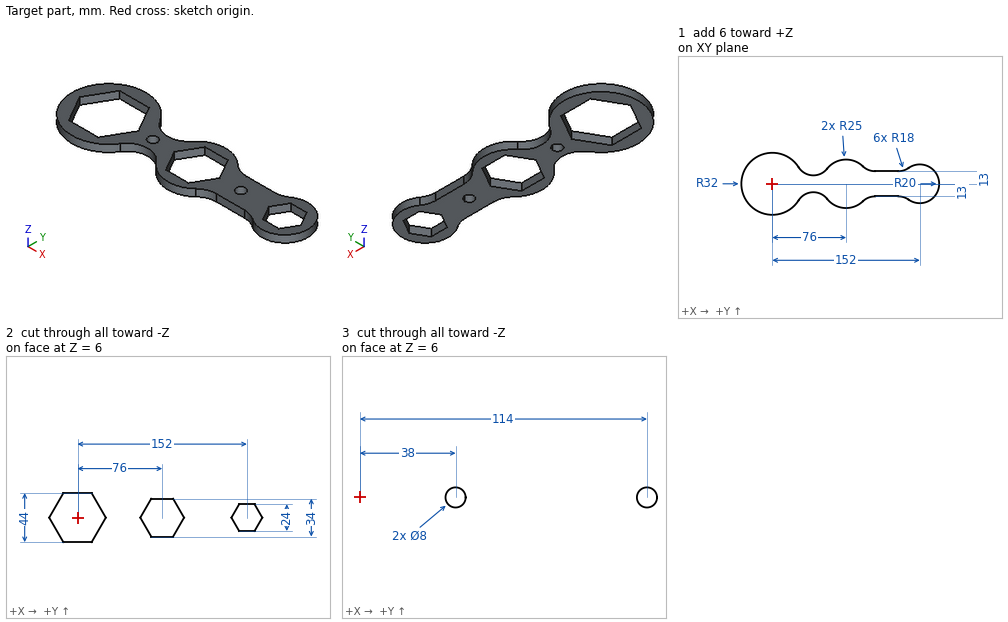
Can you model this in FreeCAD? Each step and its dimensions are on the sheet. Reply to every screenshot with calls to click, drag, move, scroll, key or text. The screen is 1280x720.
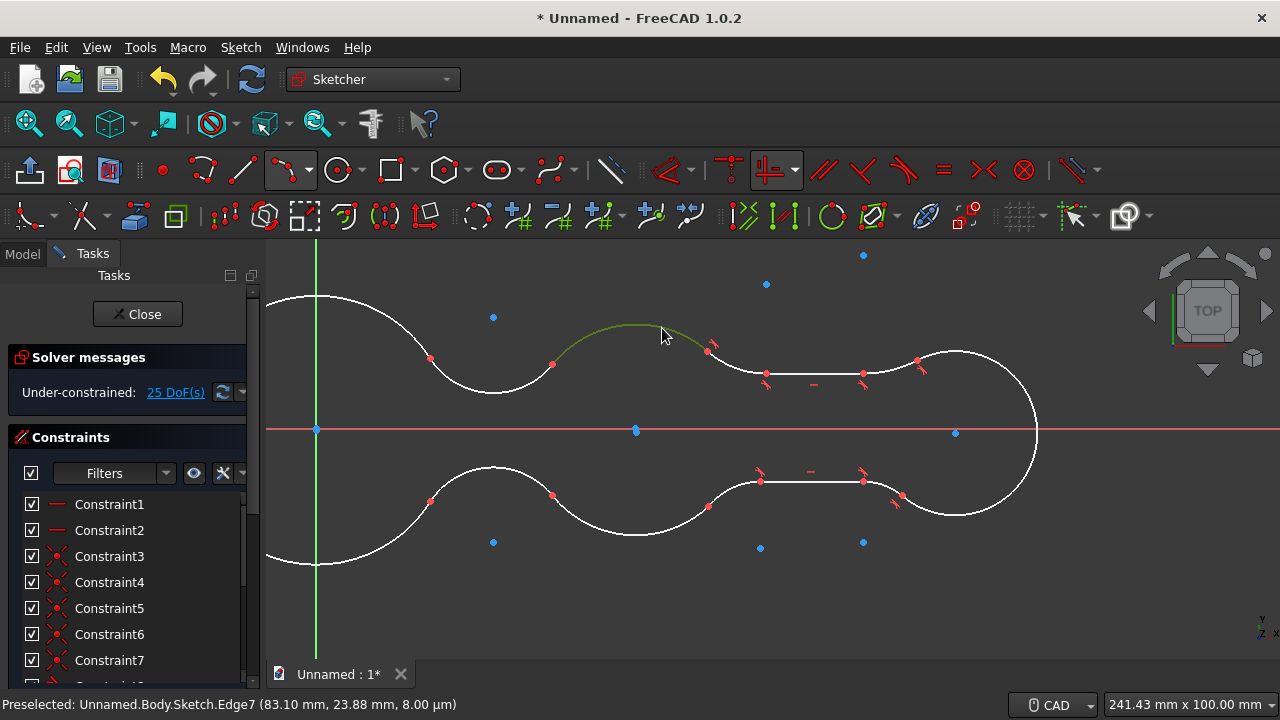
click(462, 386)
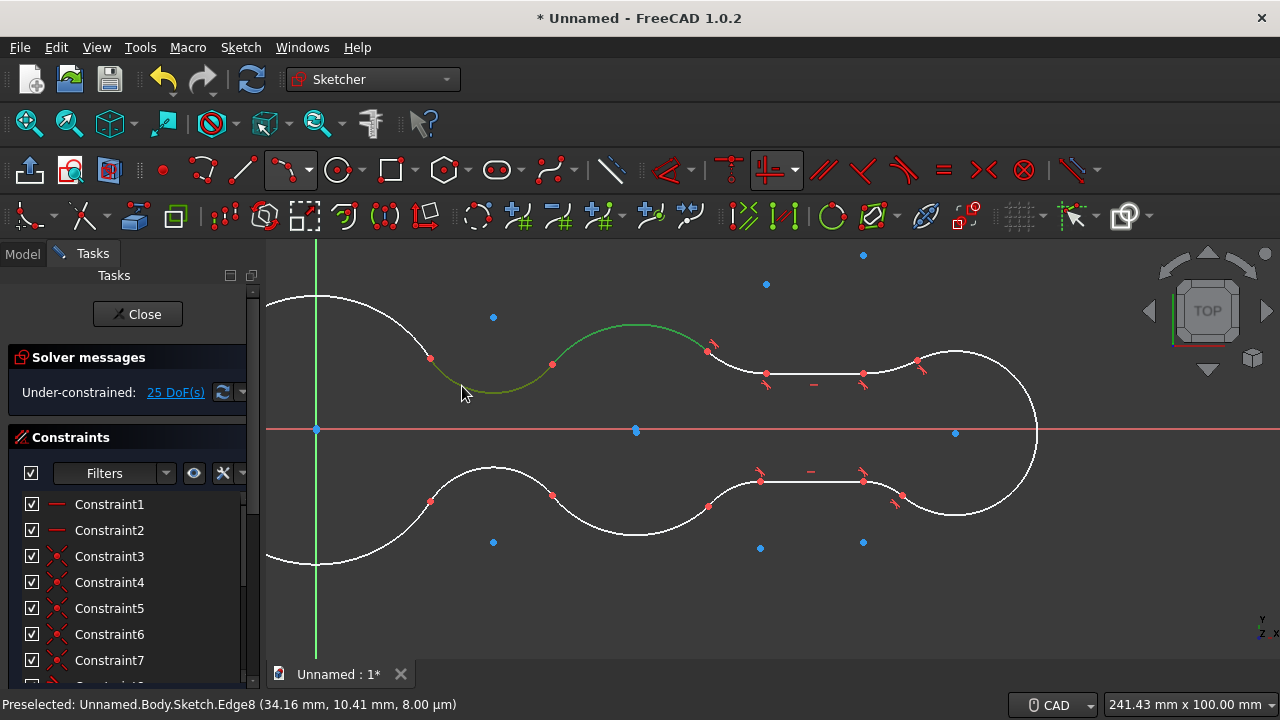
click(904, 170)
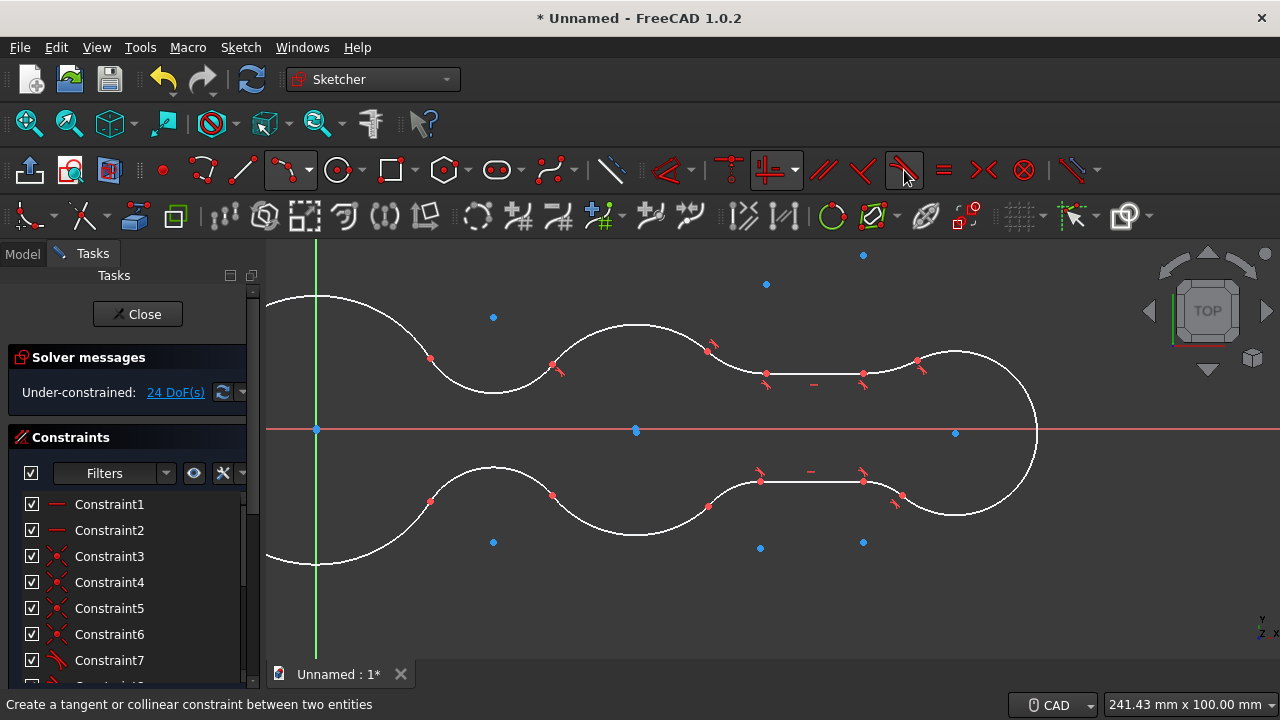
click(462, 386)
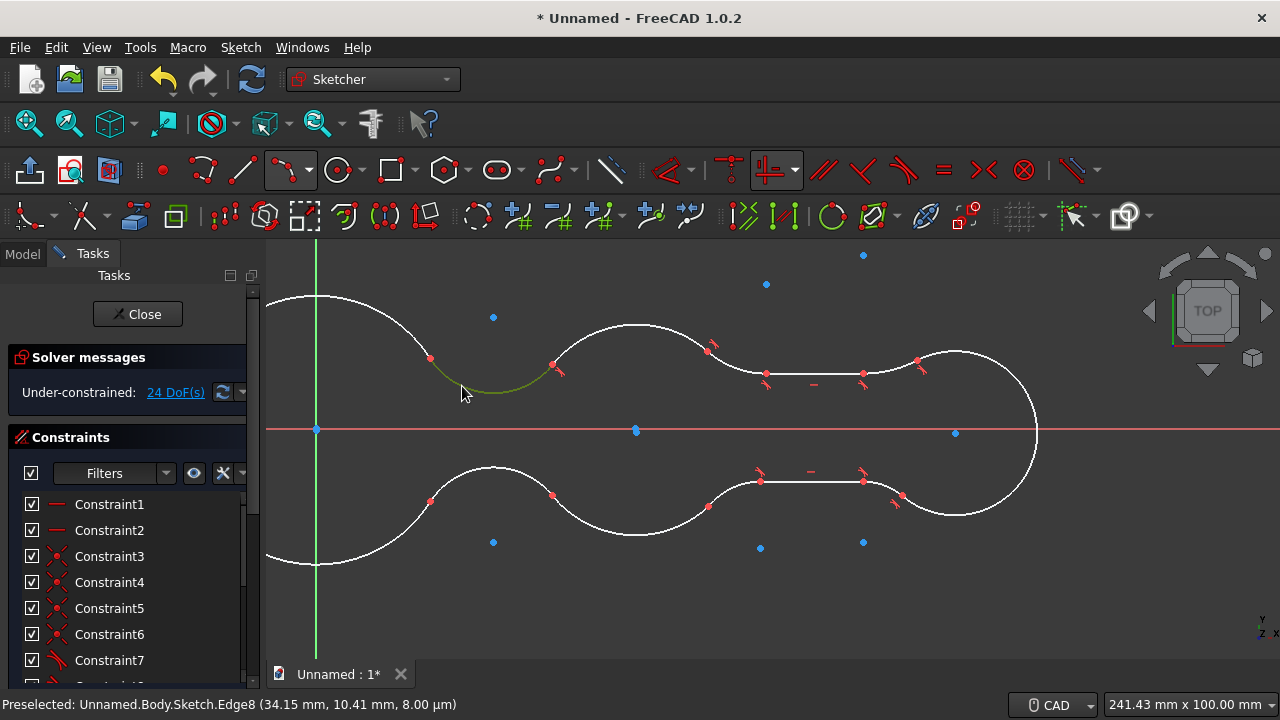
click(313, 296)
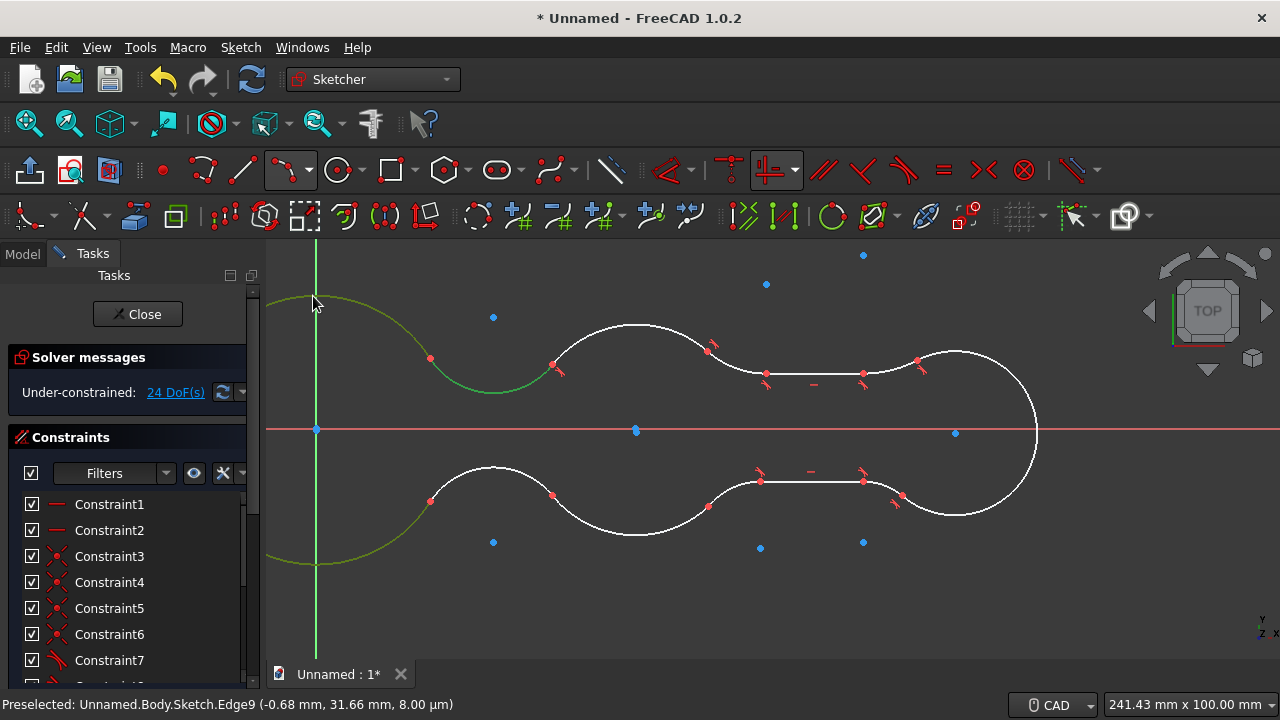
click(904, 170)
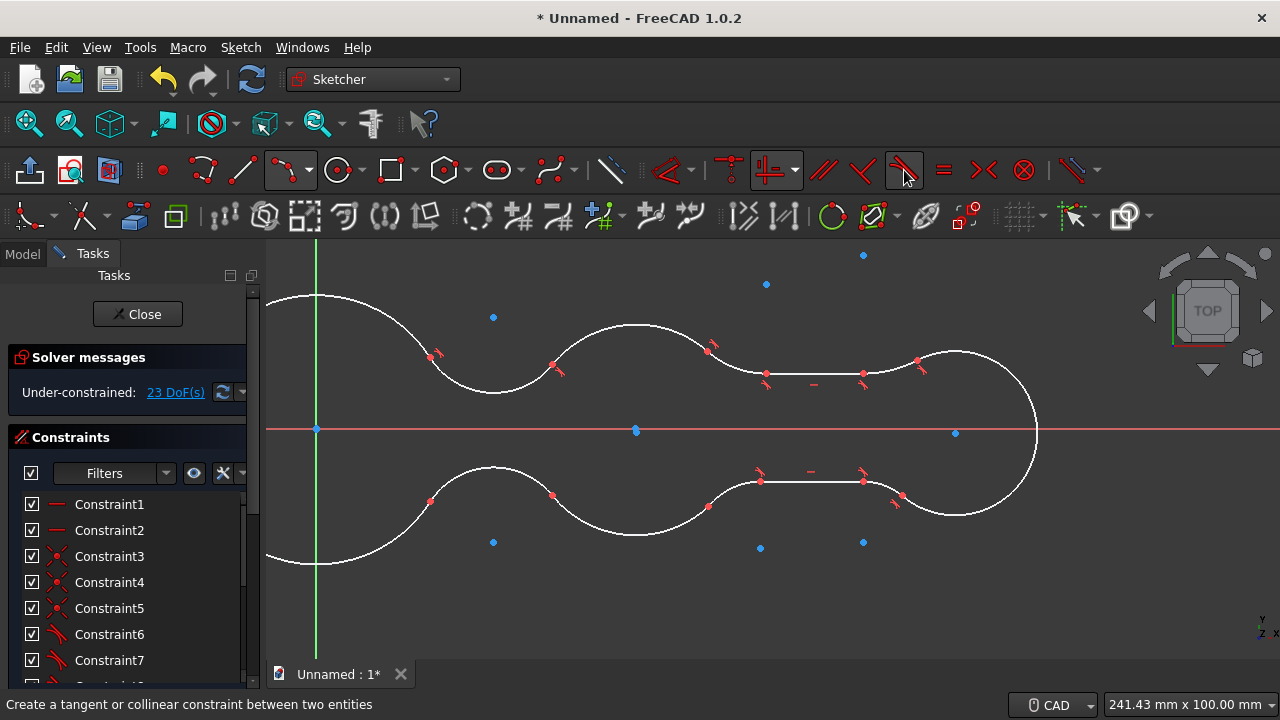
click(313, 295)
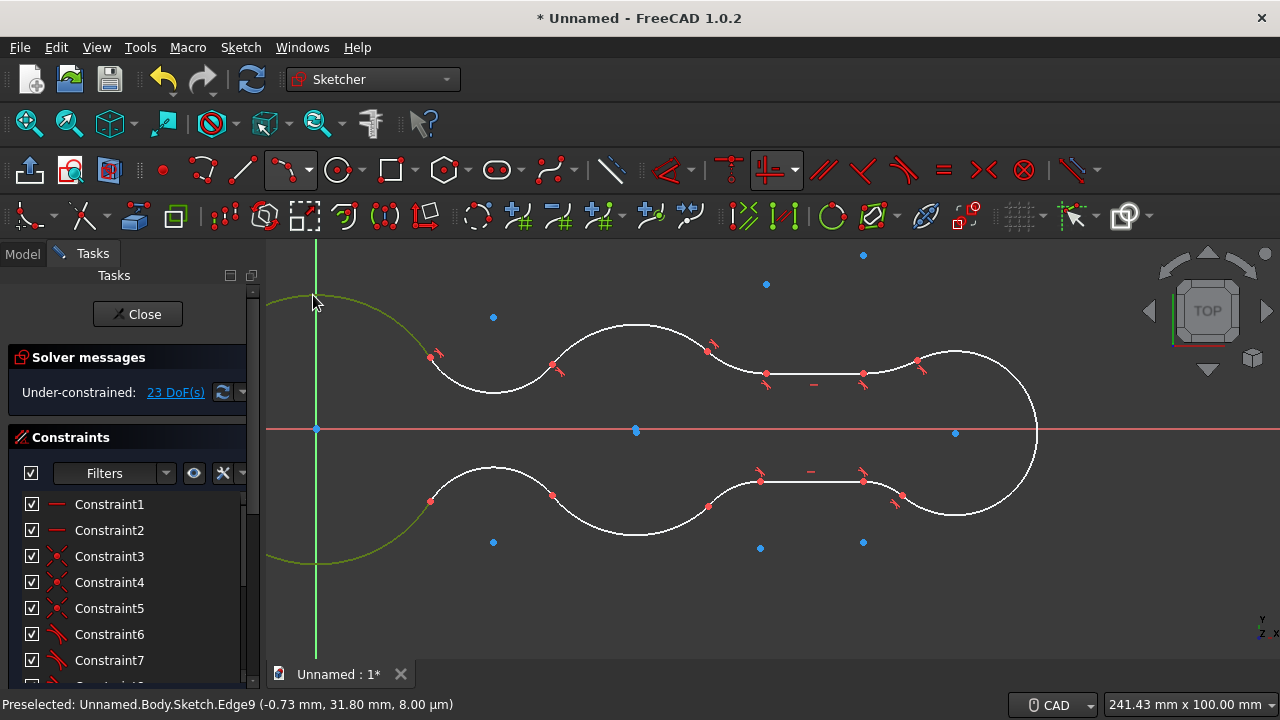
click(518, 472)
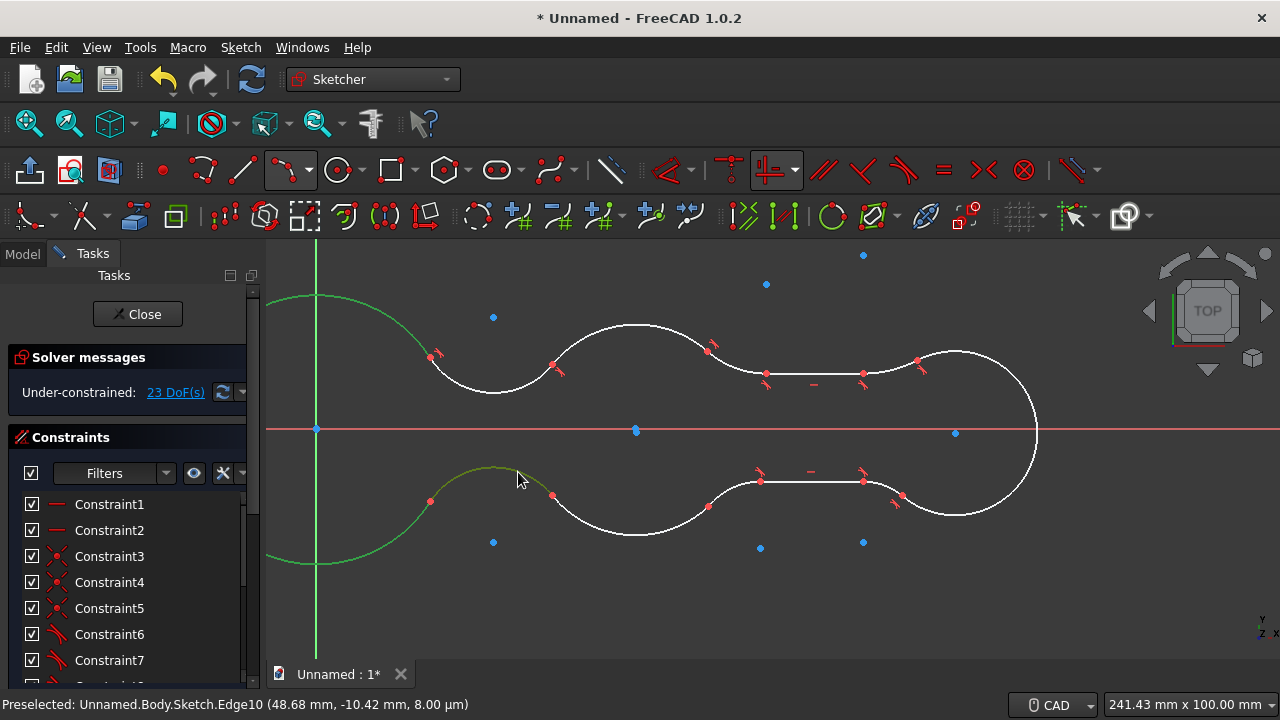
click(904, 170)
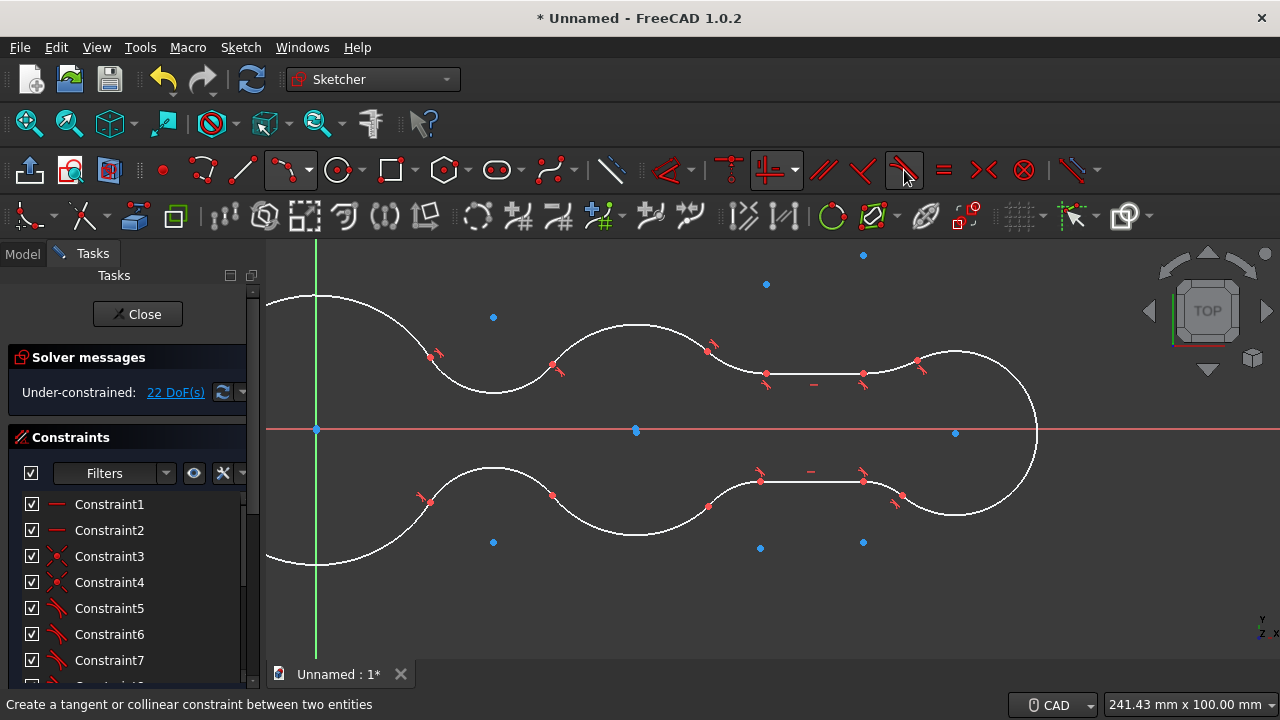
click(518, 472)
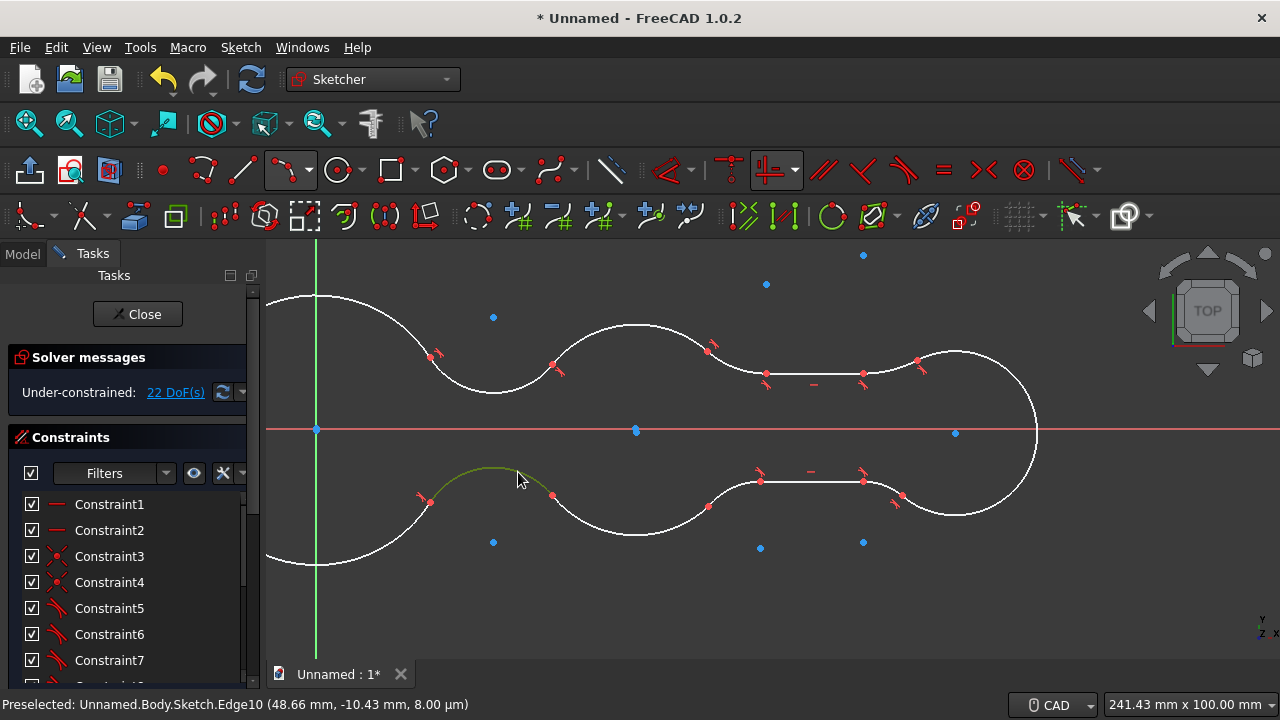
click(594, 527)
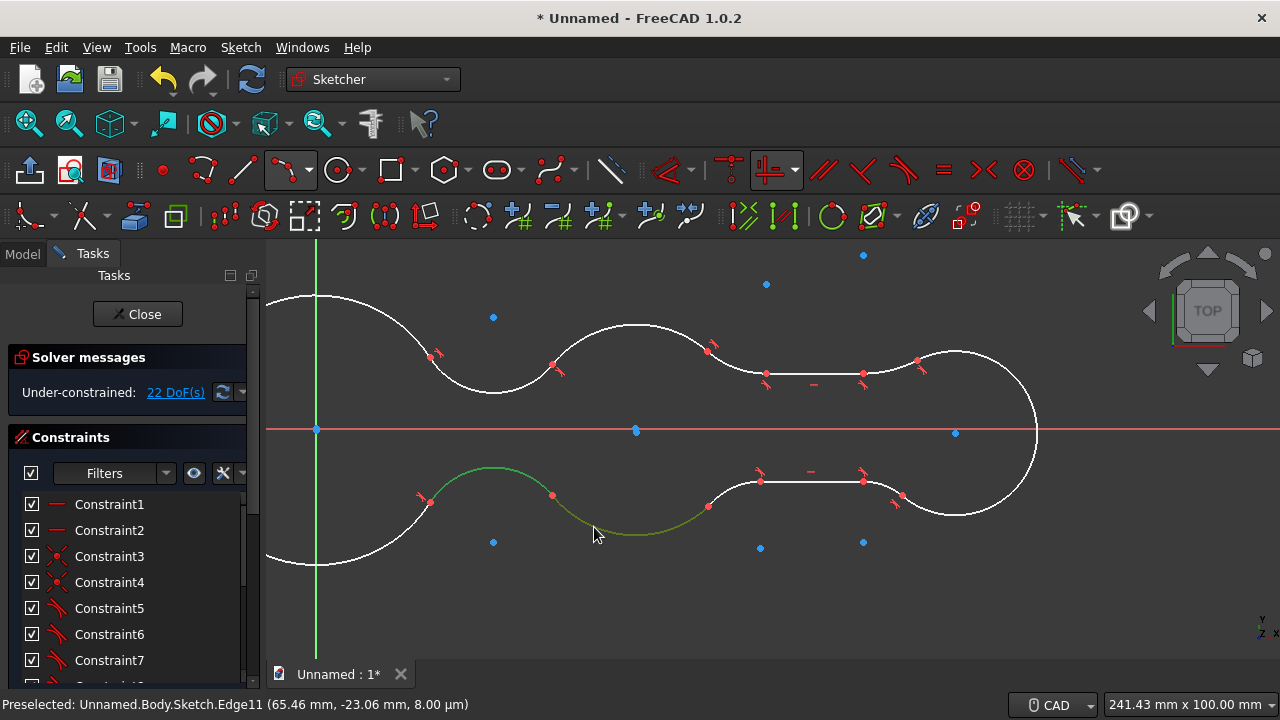
click(904, 170)